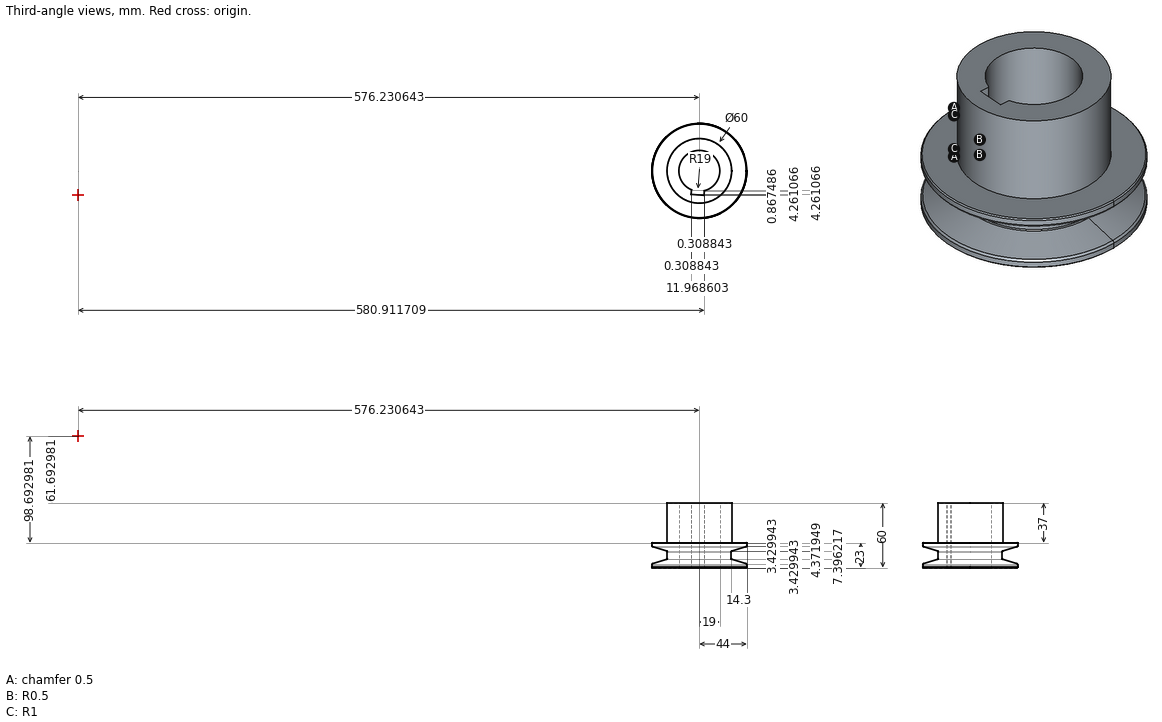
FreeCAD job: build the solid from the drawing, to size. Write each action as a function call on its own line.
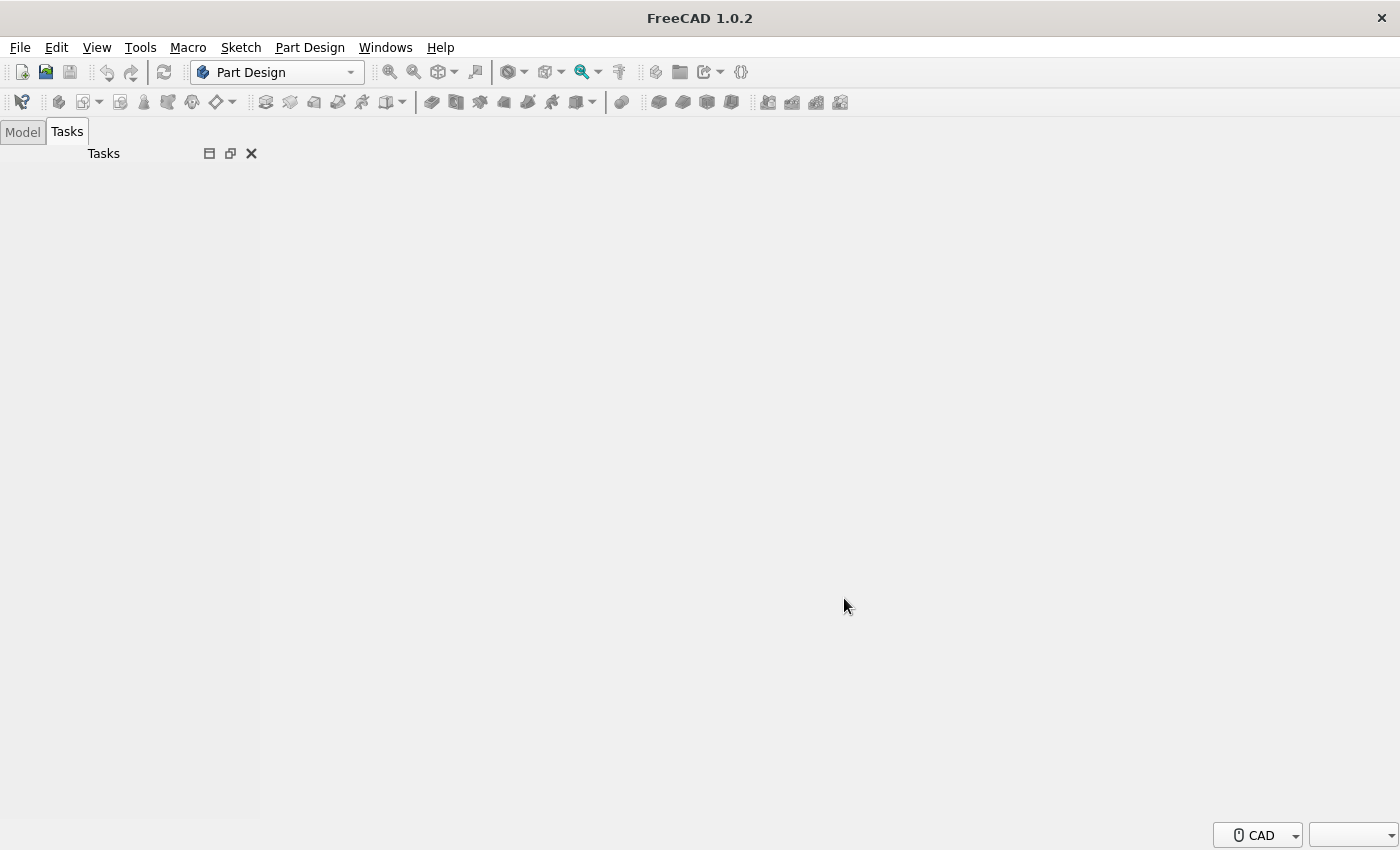
click(22, 72)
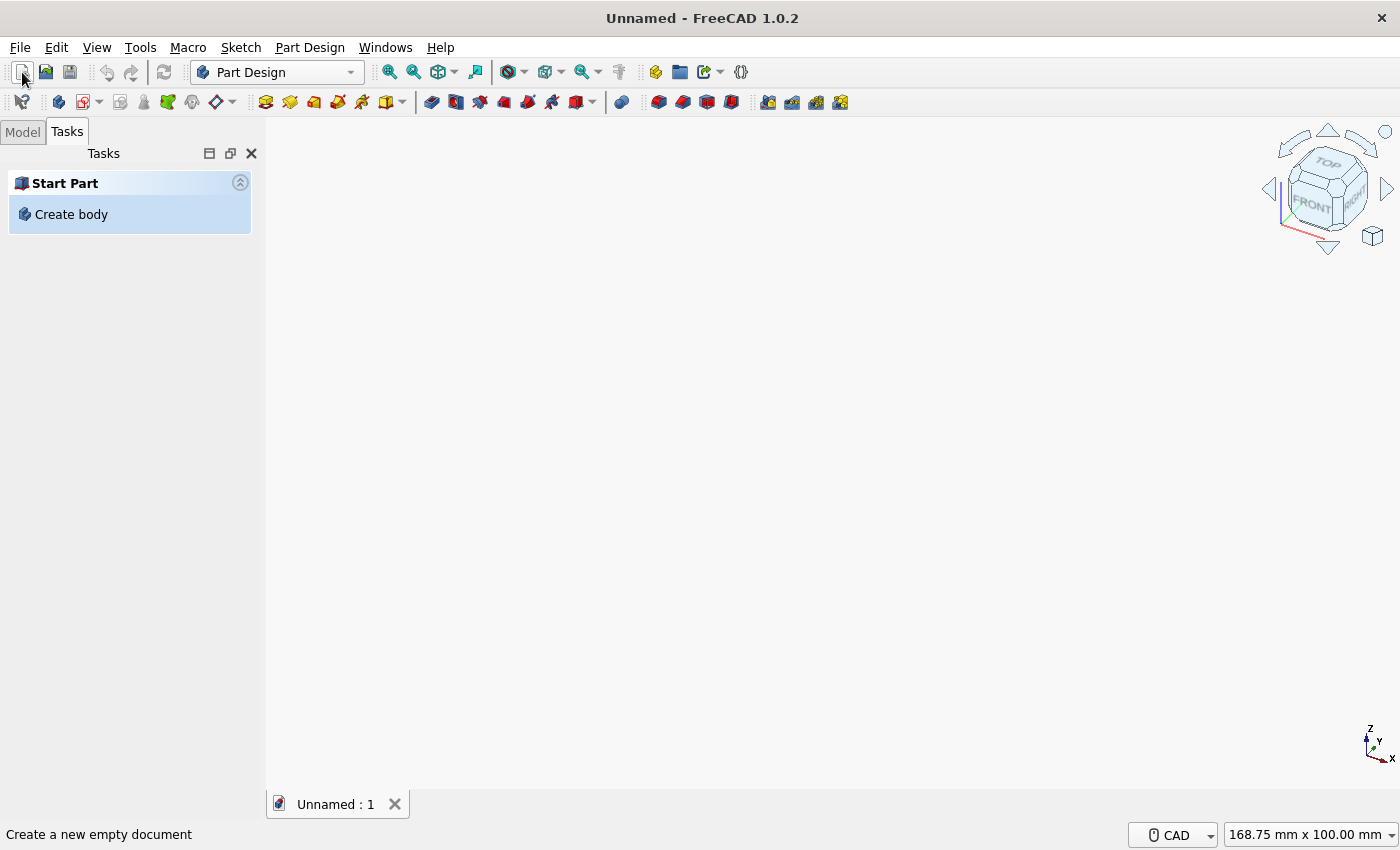
click(60, 102)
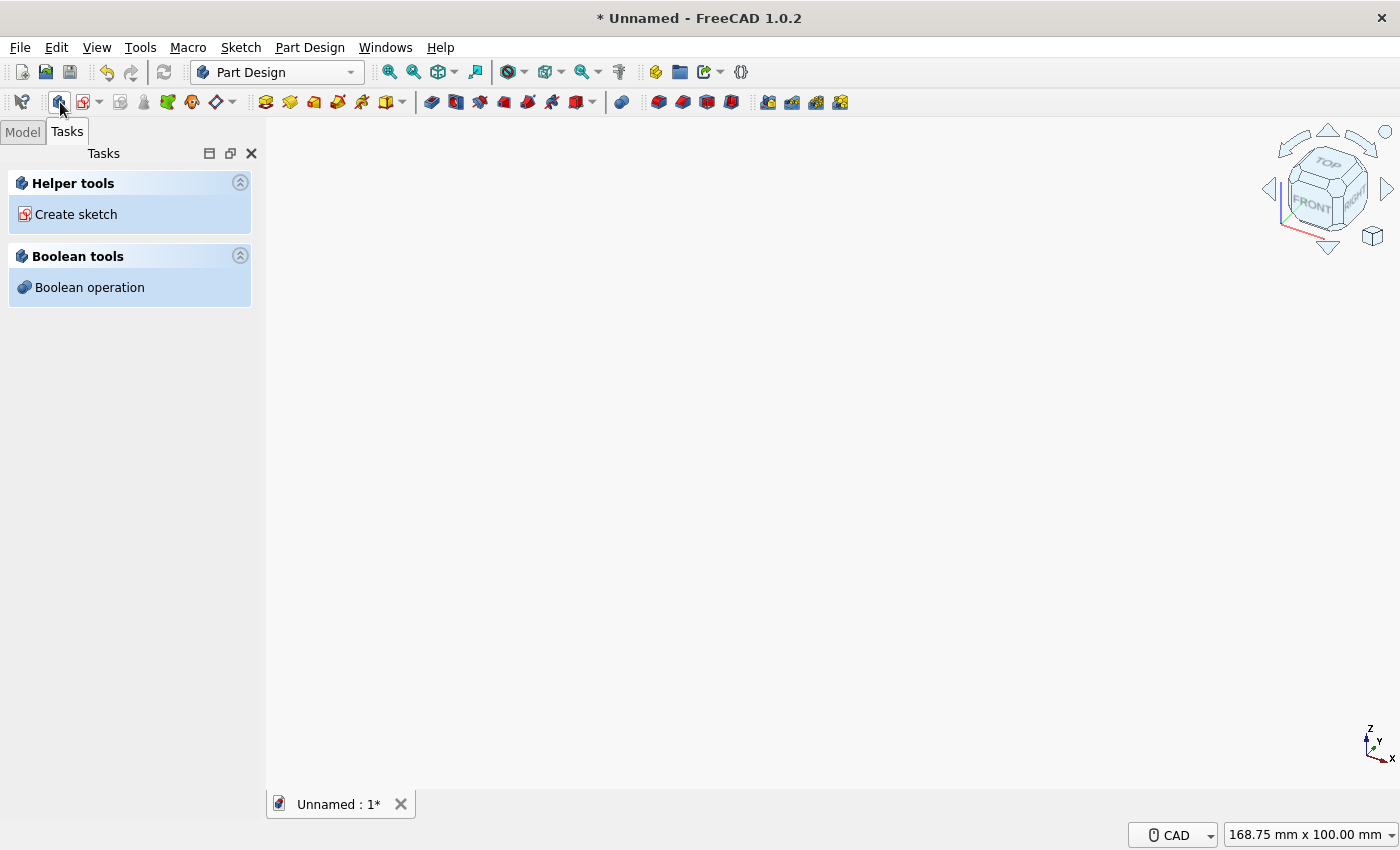
click(23, 131)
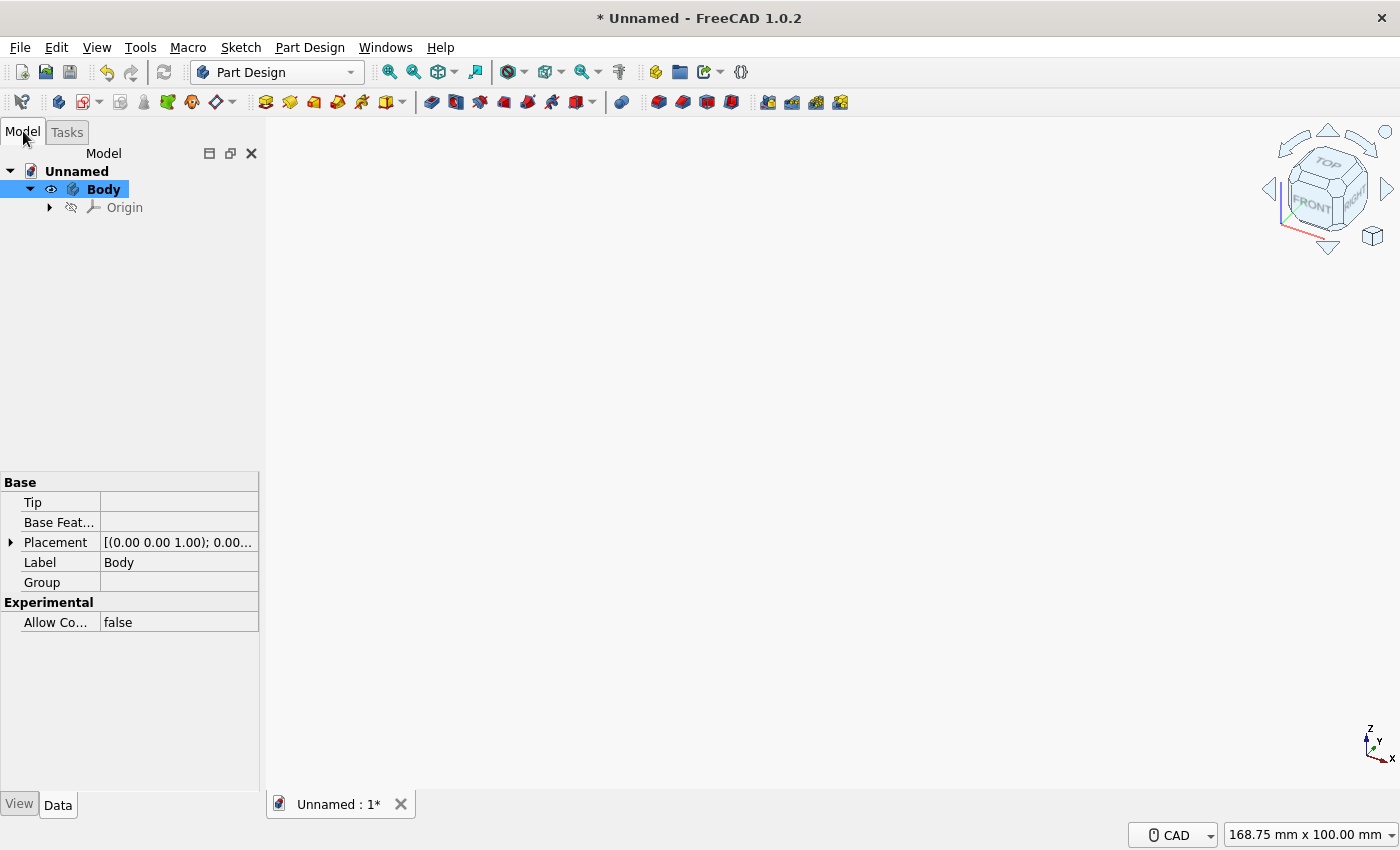
click(50, 207)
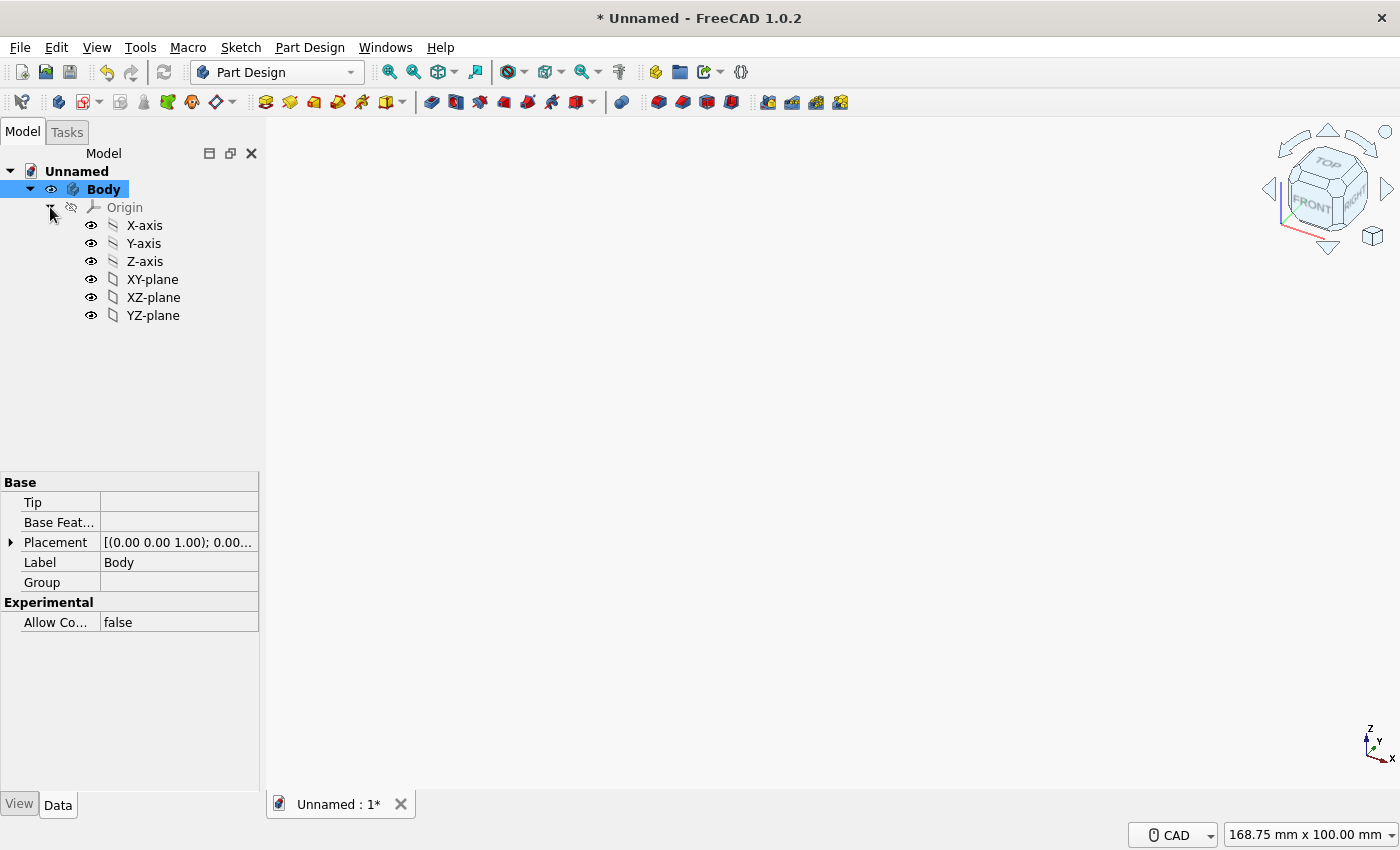
click(136, 297)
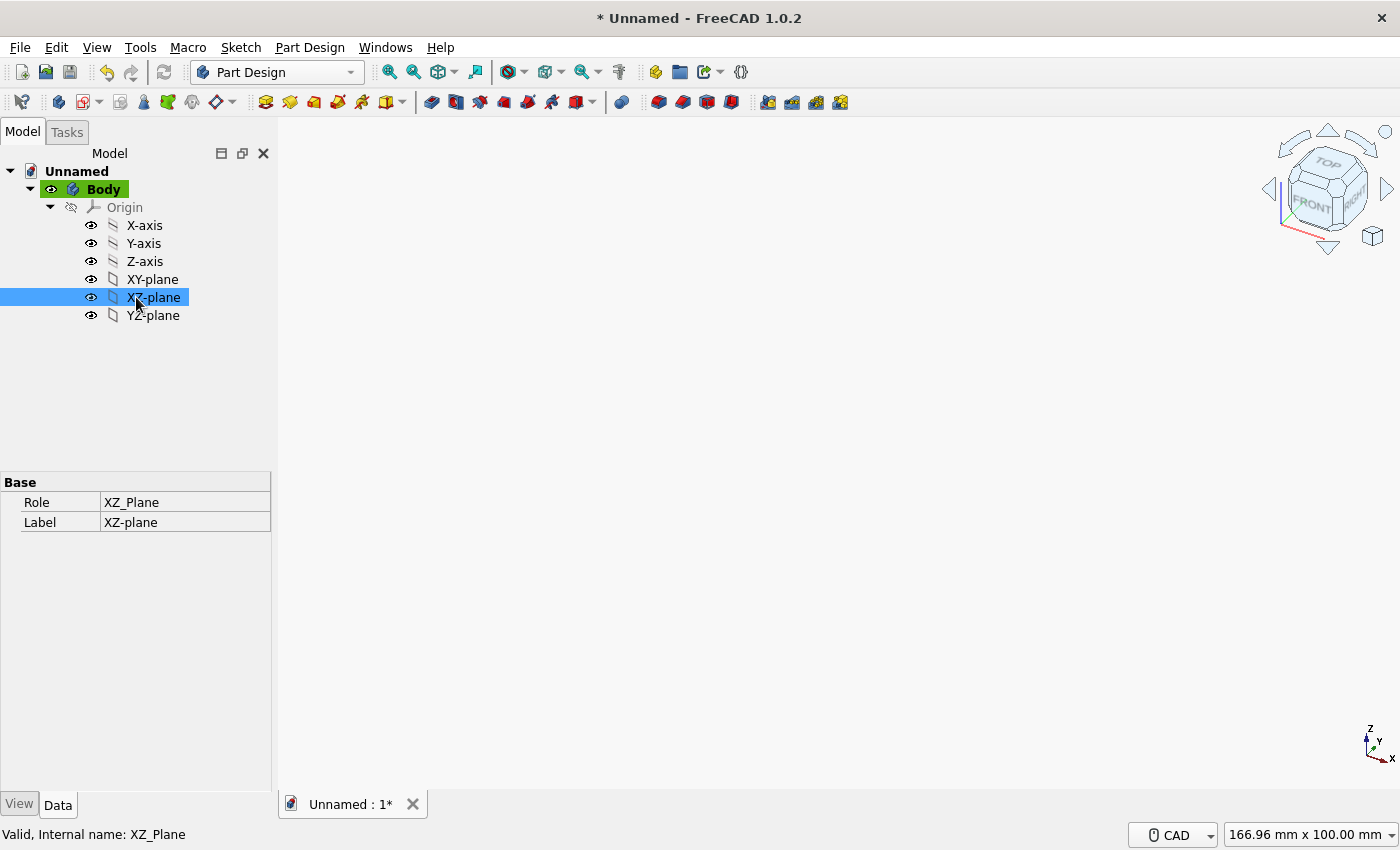
click(216, 102)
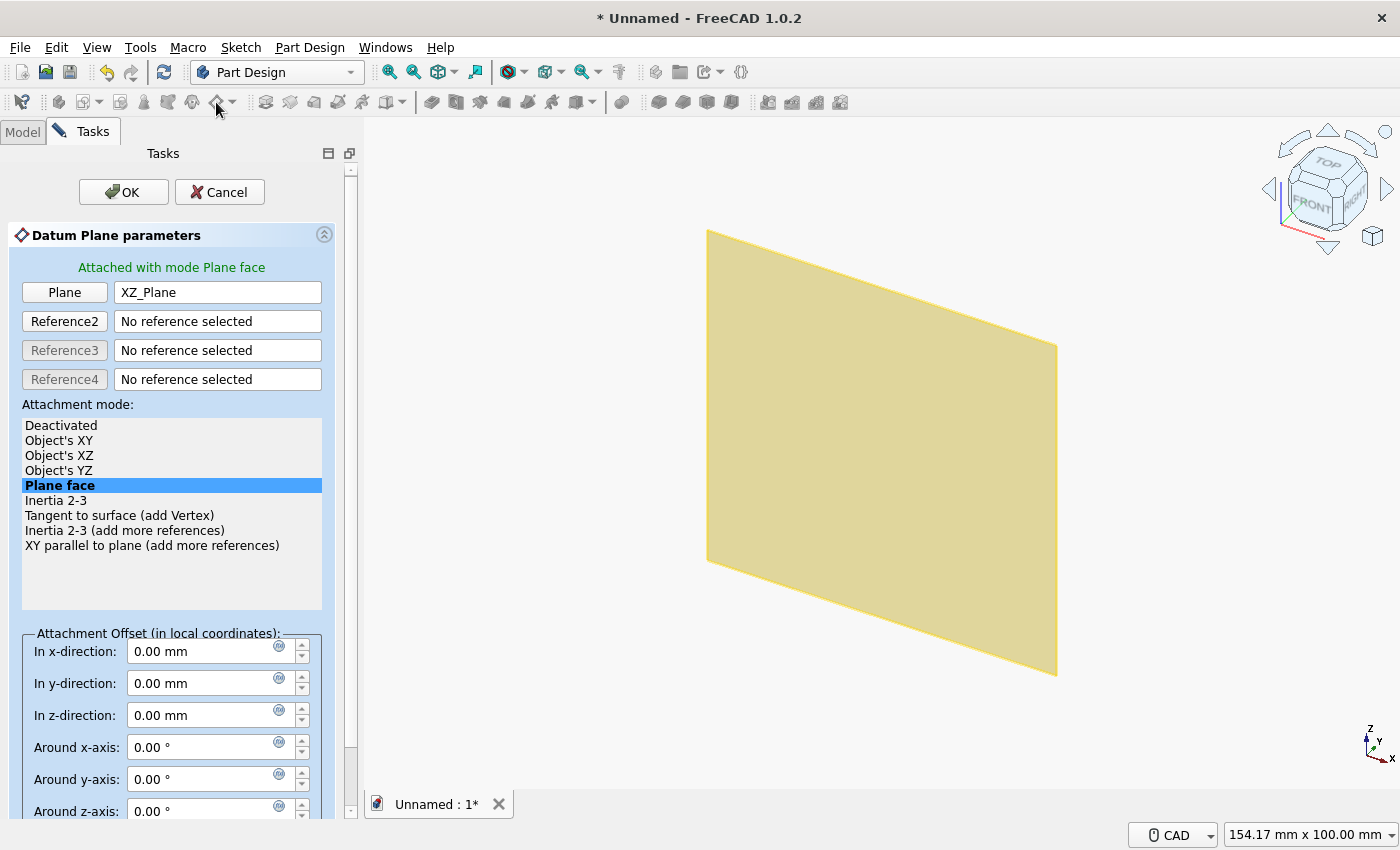
triple_click(210, 715)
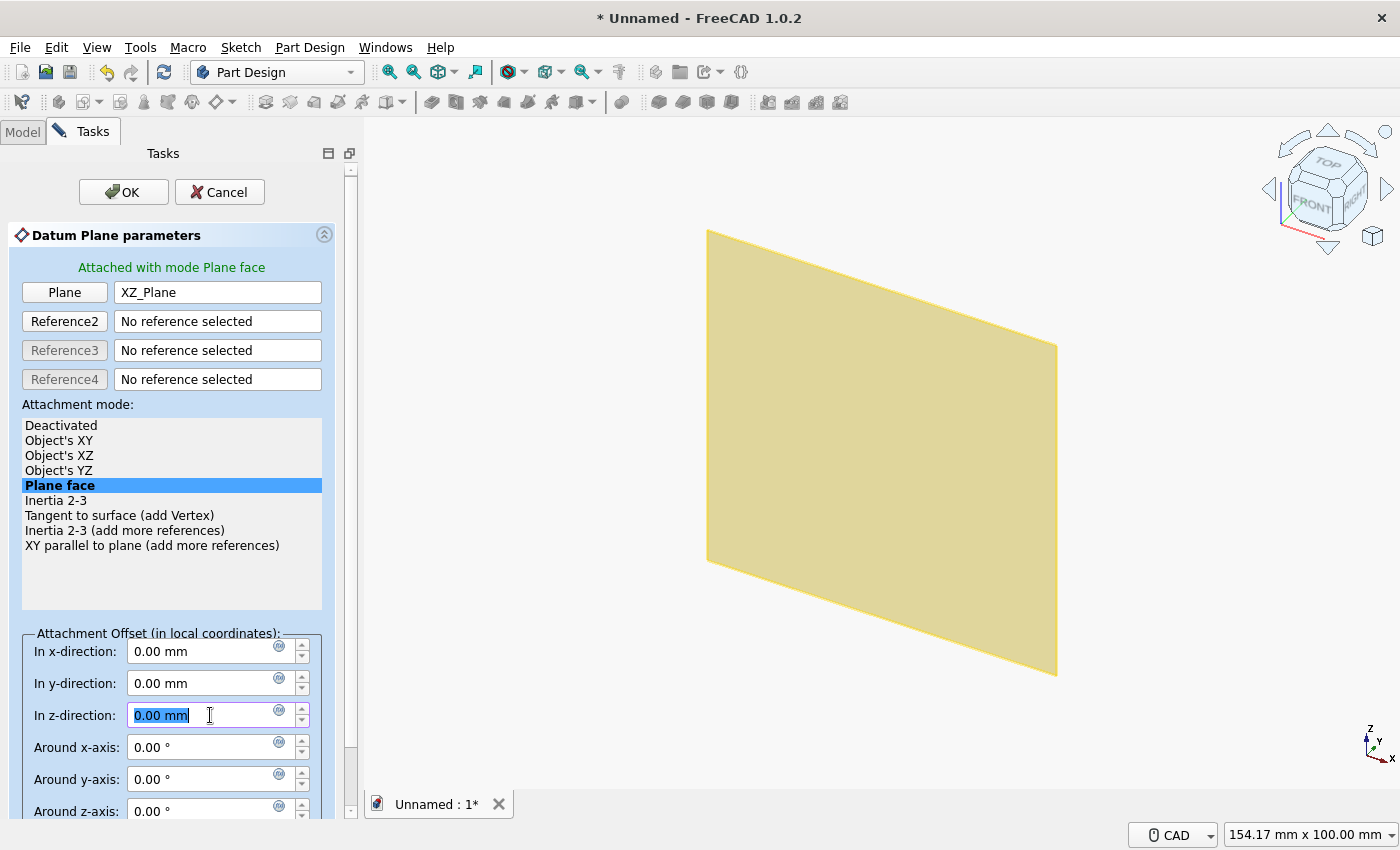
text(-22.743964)
key(Tab)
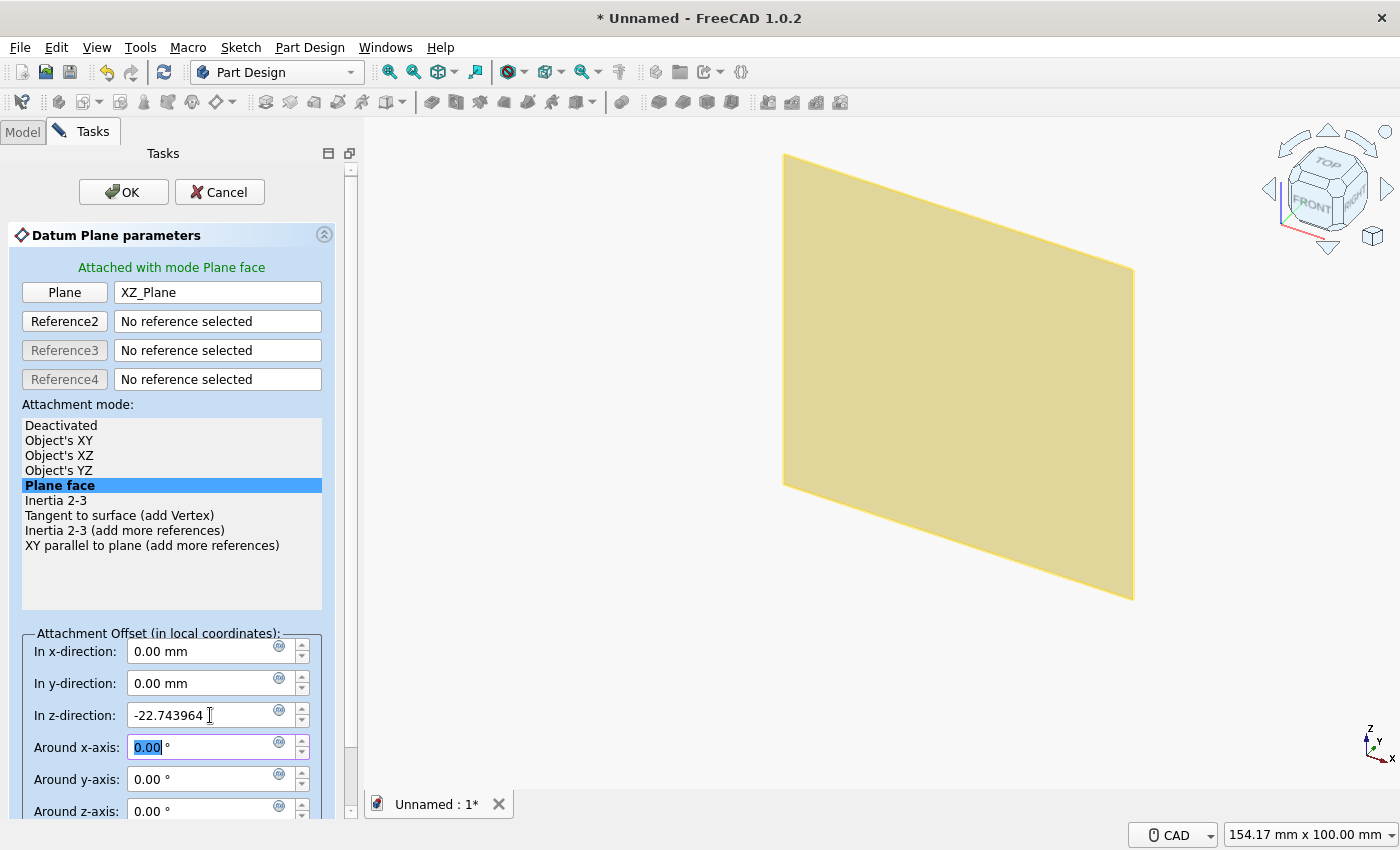
click(124, 192)